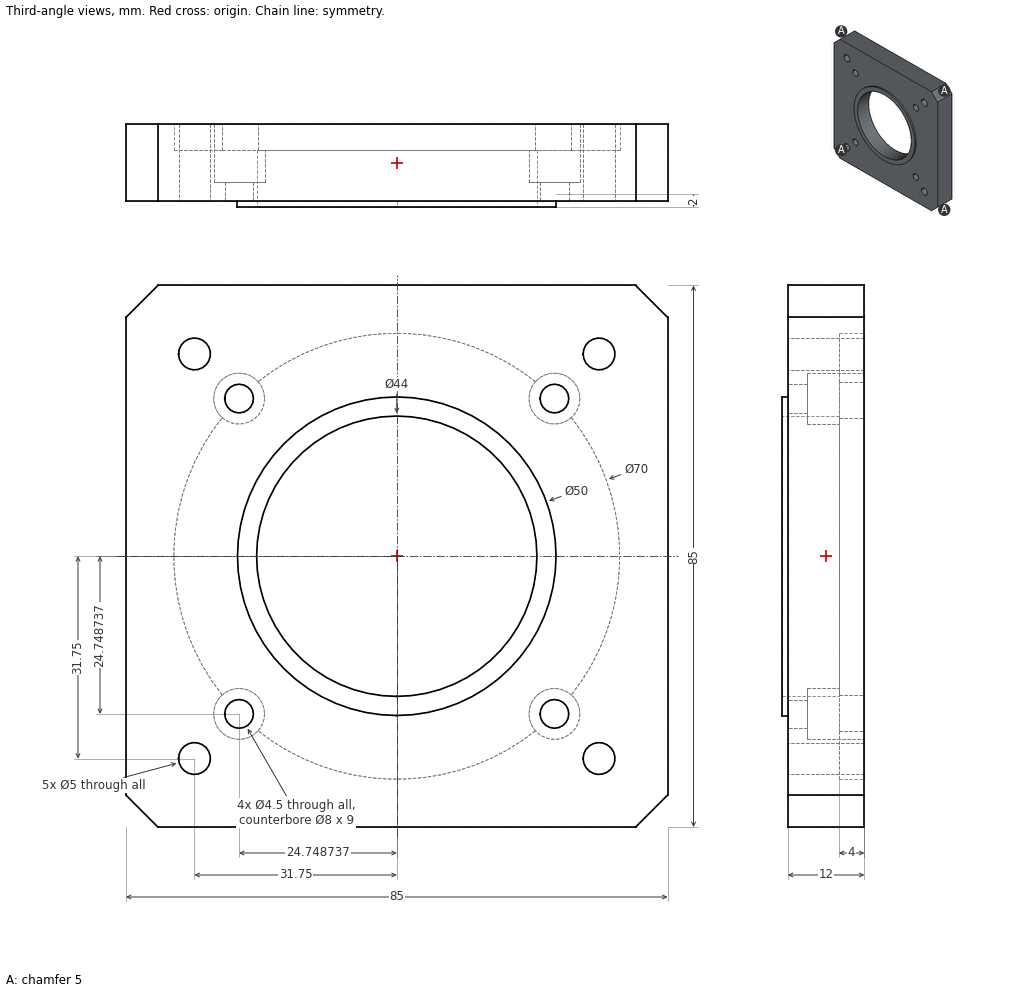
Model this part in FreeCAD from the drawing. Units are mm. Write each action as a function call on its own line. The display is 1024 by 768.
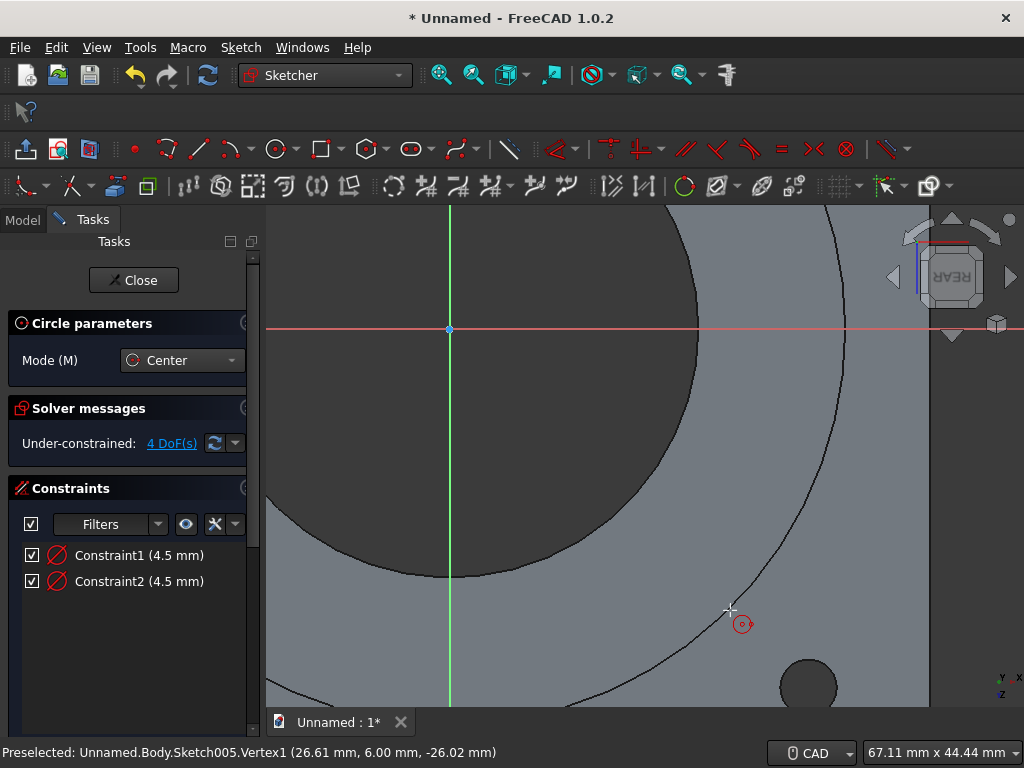
click(730, 609)
move(747, 591)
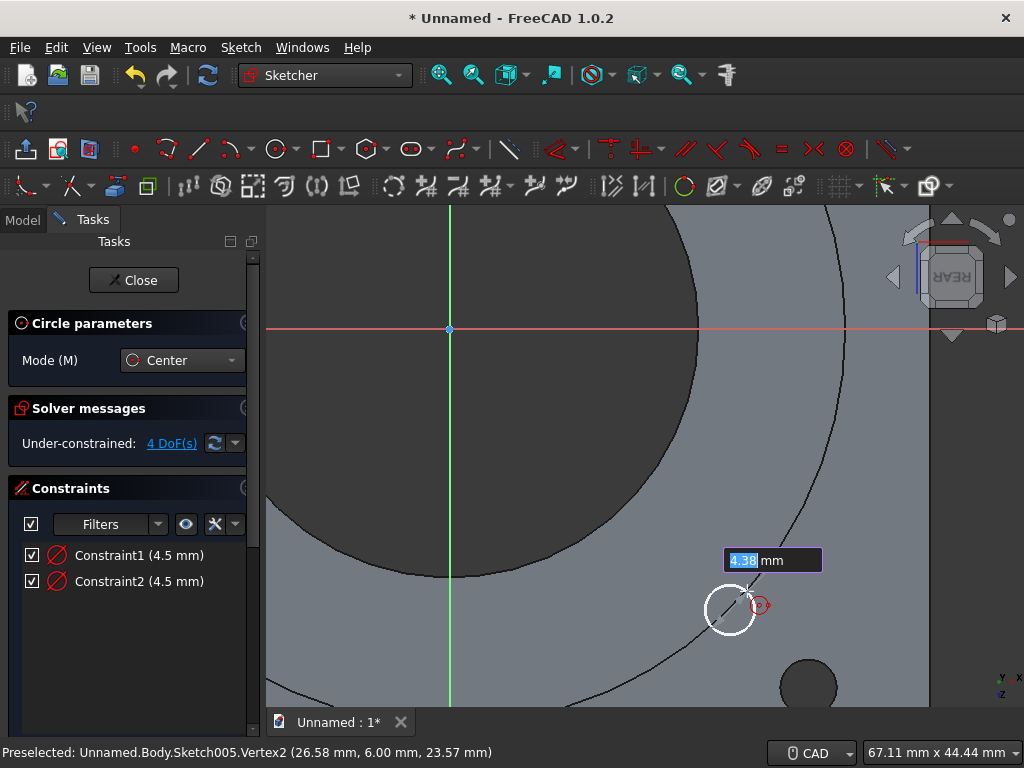
text(4.5)
key(Return)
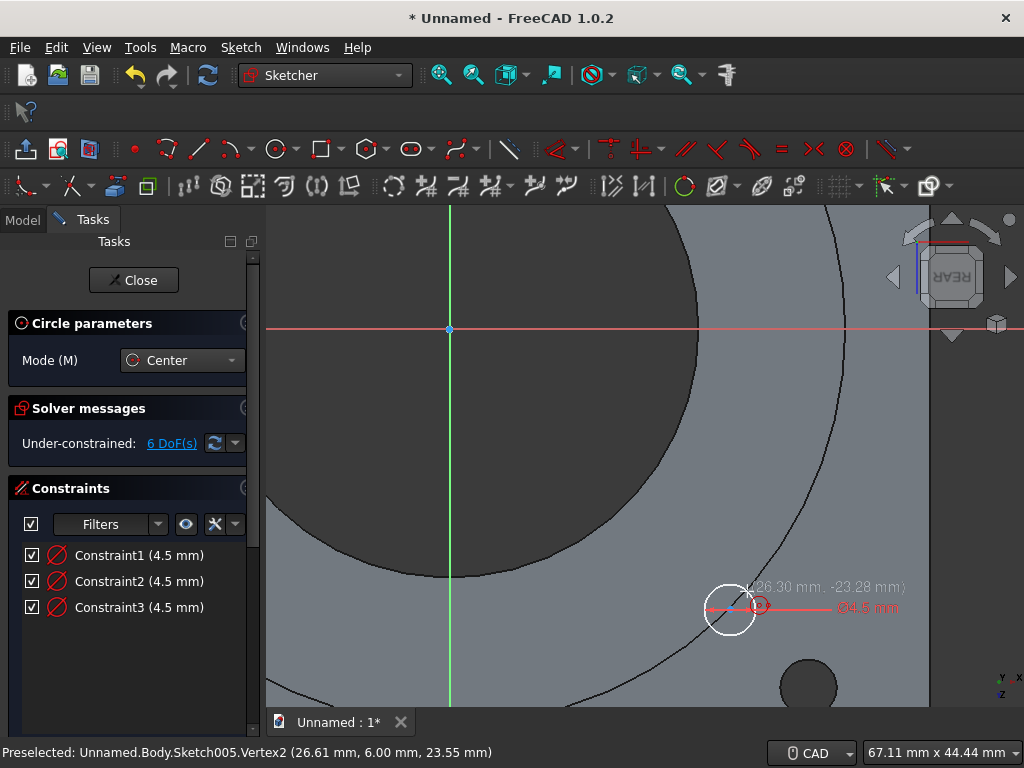
scroll(730, 610, down, 3)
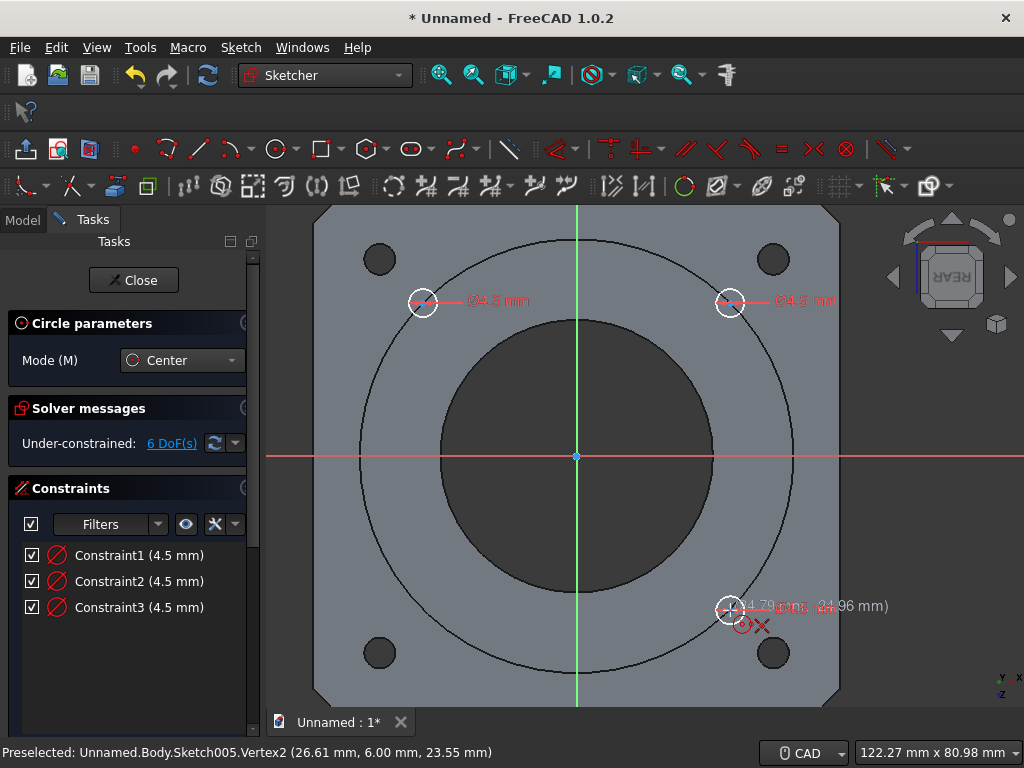
scroll(423, 610, up, 3)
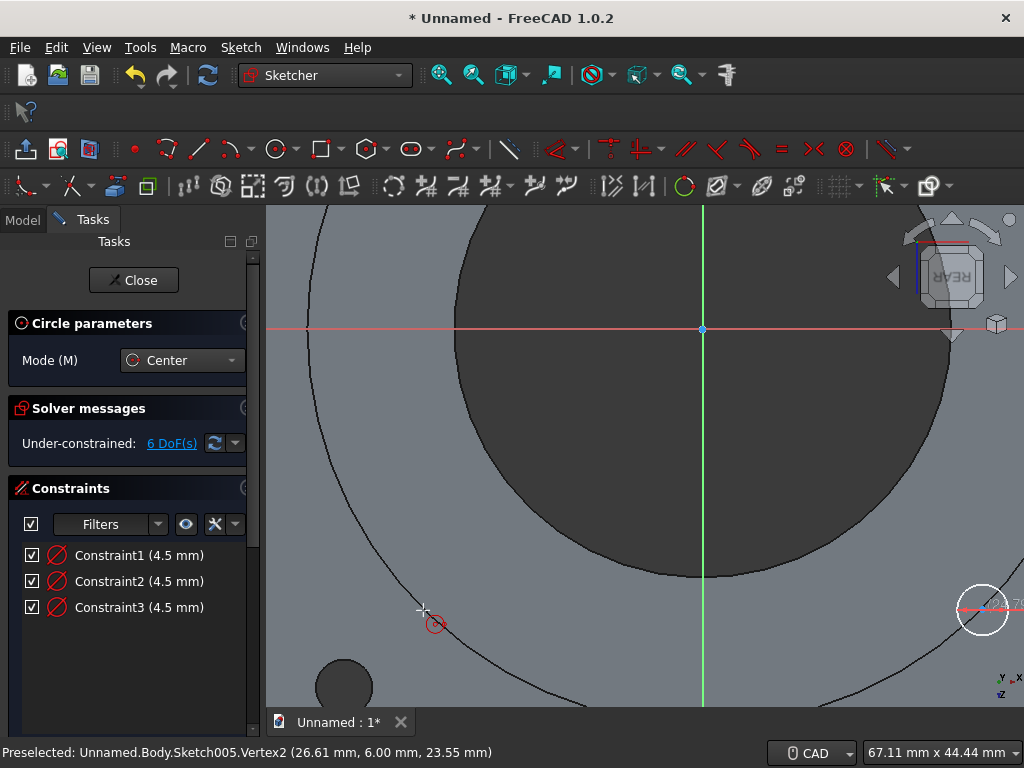
click(423, 609)
move(441, 591)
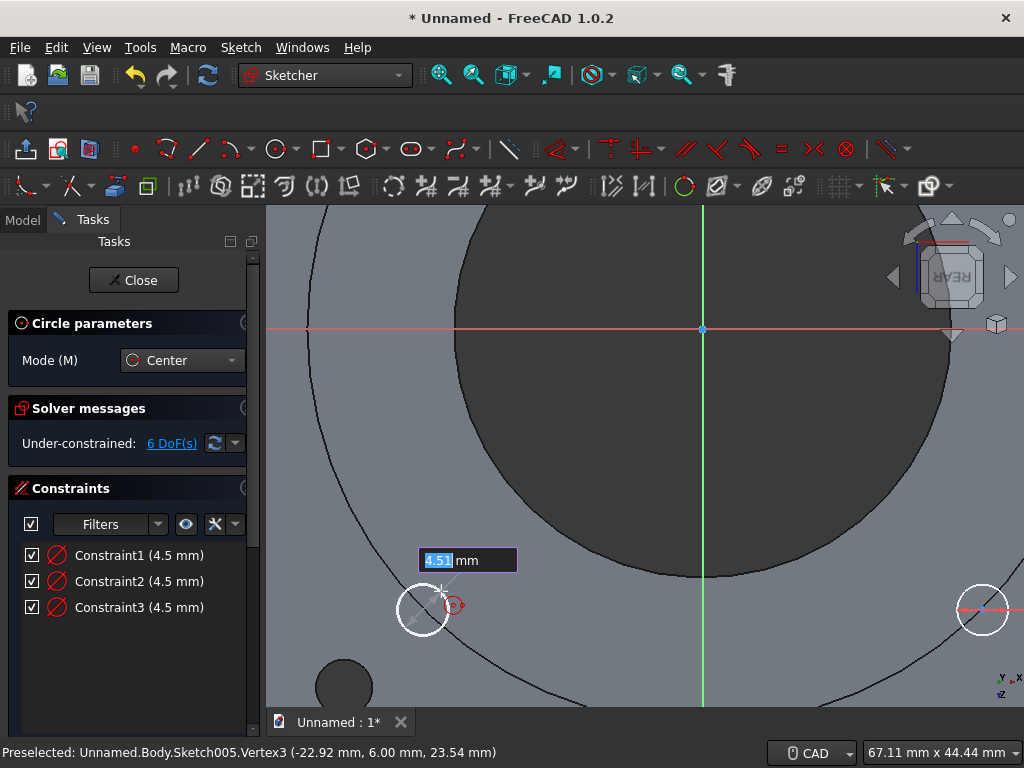
text(4.5)
key(Return)
key(Escape)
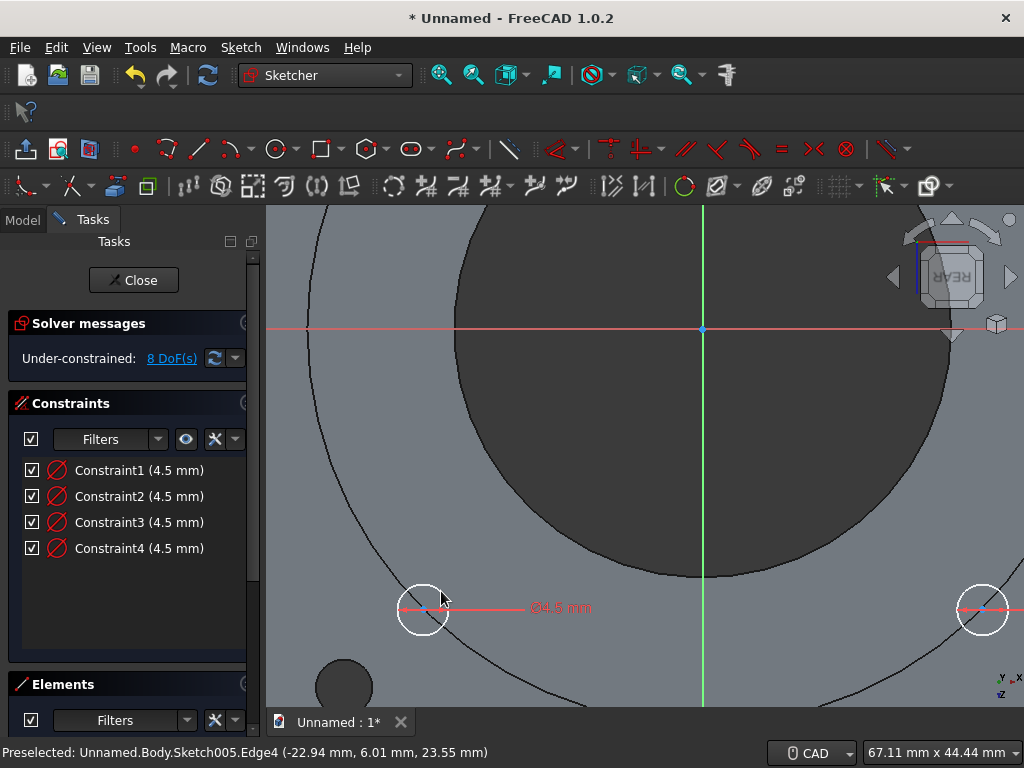
scroll(423, 610, down, 3)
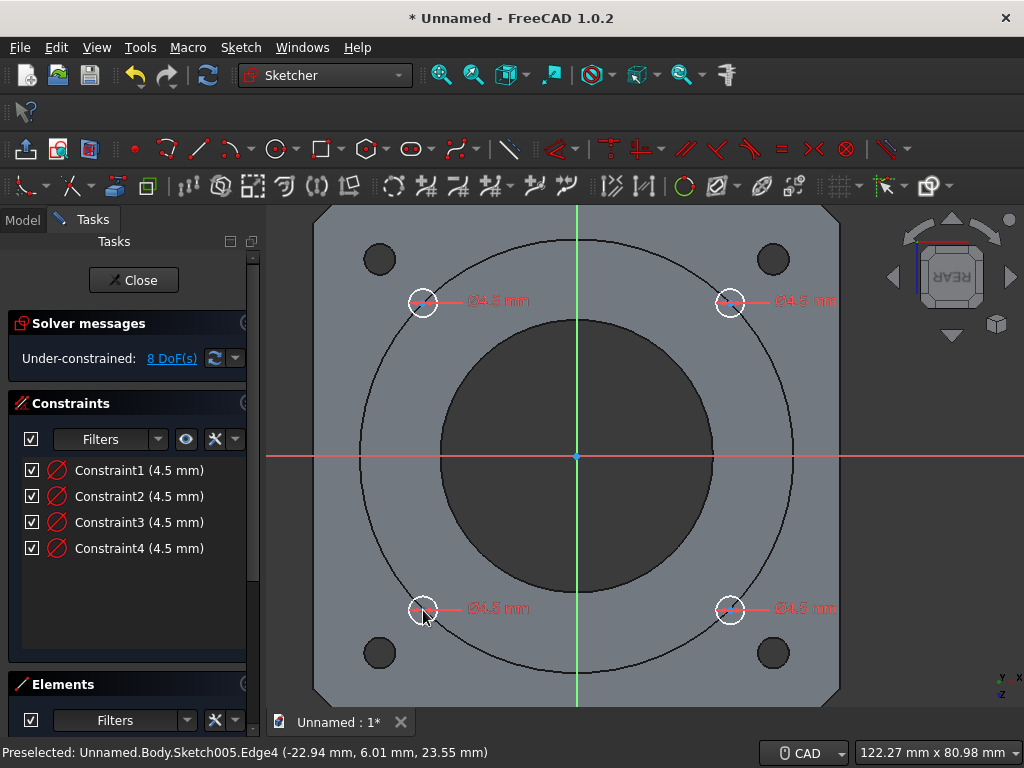
click(423, 303)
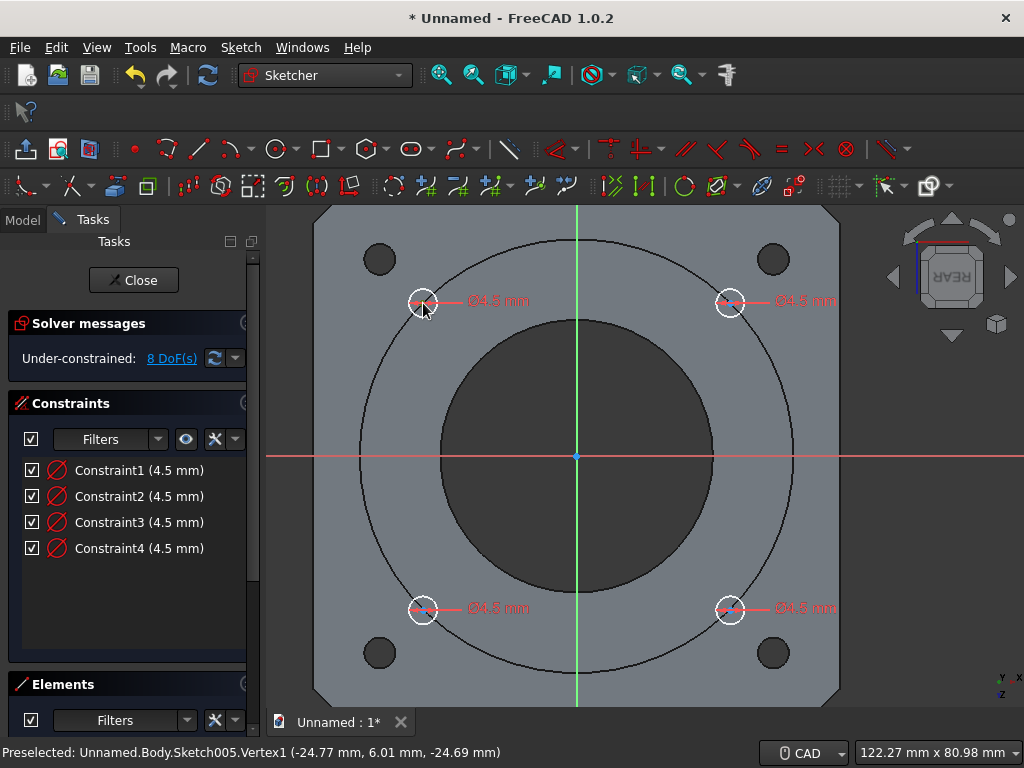
click(730, 303)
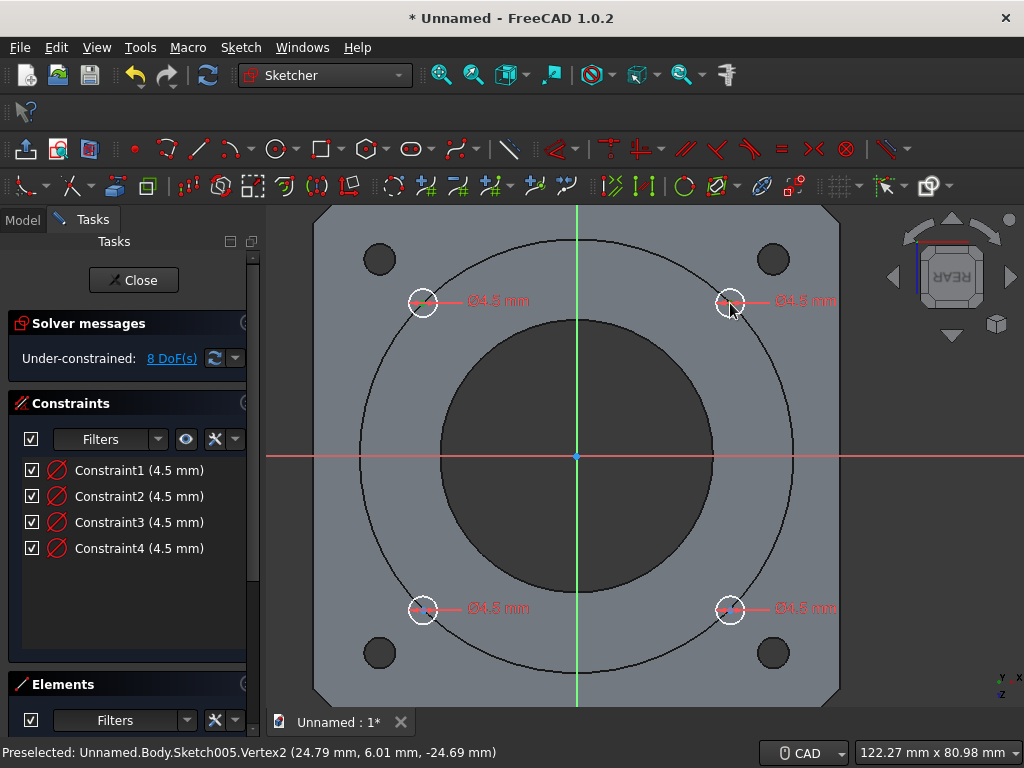
click(577, 647)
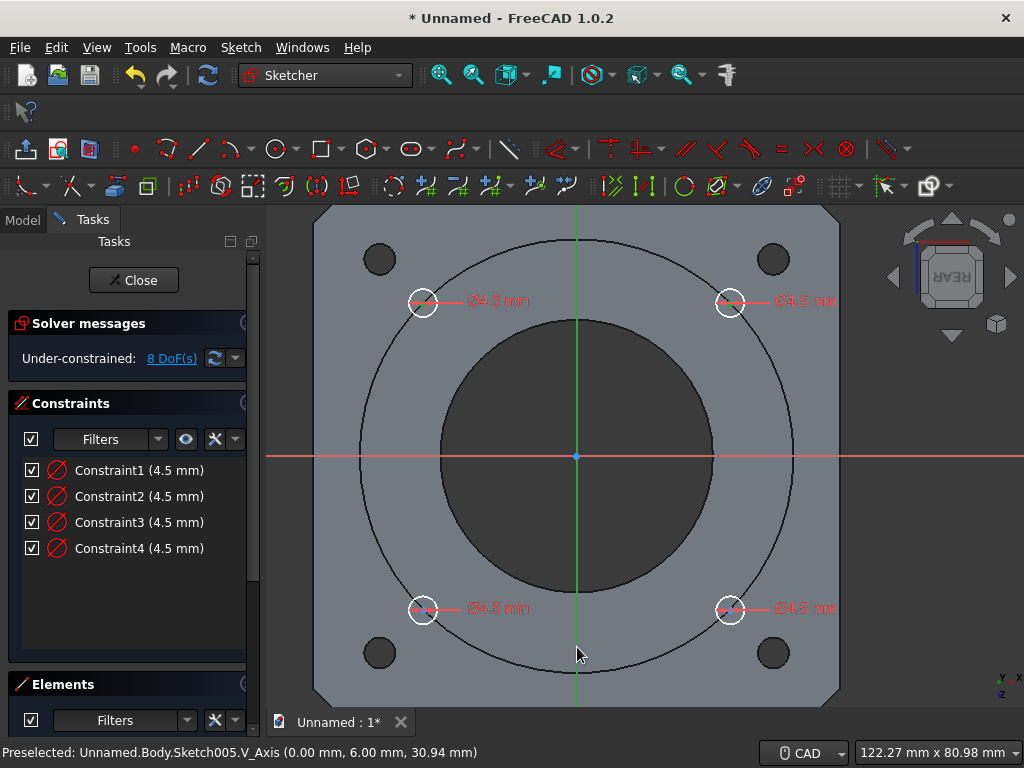
key(s)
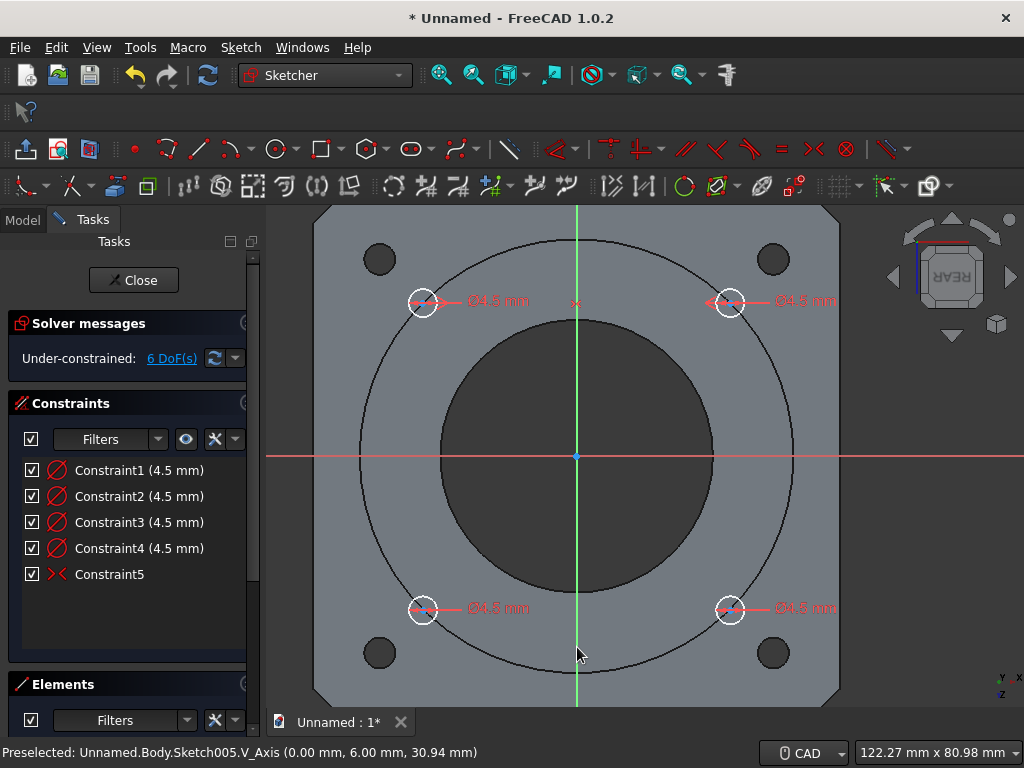
click(730, 303)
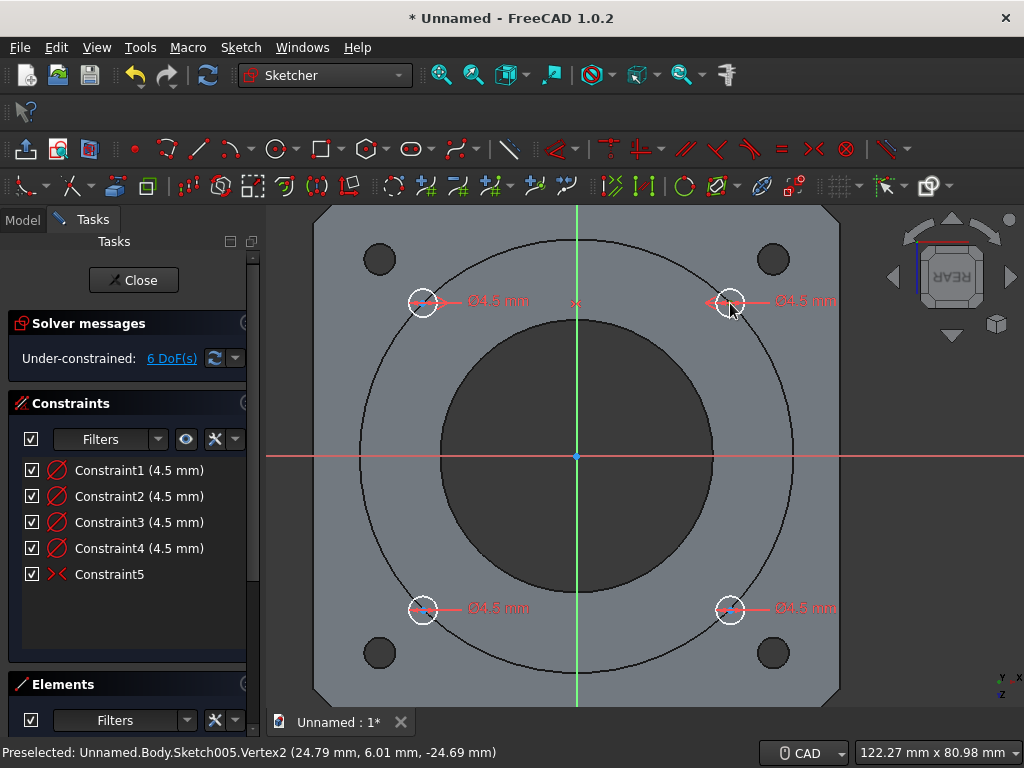
click(730, 610)